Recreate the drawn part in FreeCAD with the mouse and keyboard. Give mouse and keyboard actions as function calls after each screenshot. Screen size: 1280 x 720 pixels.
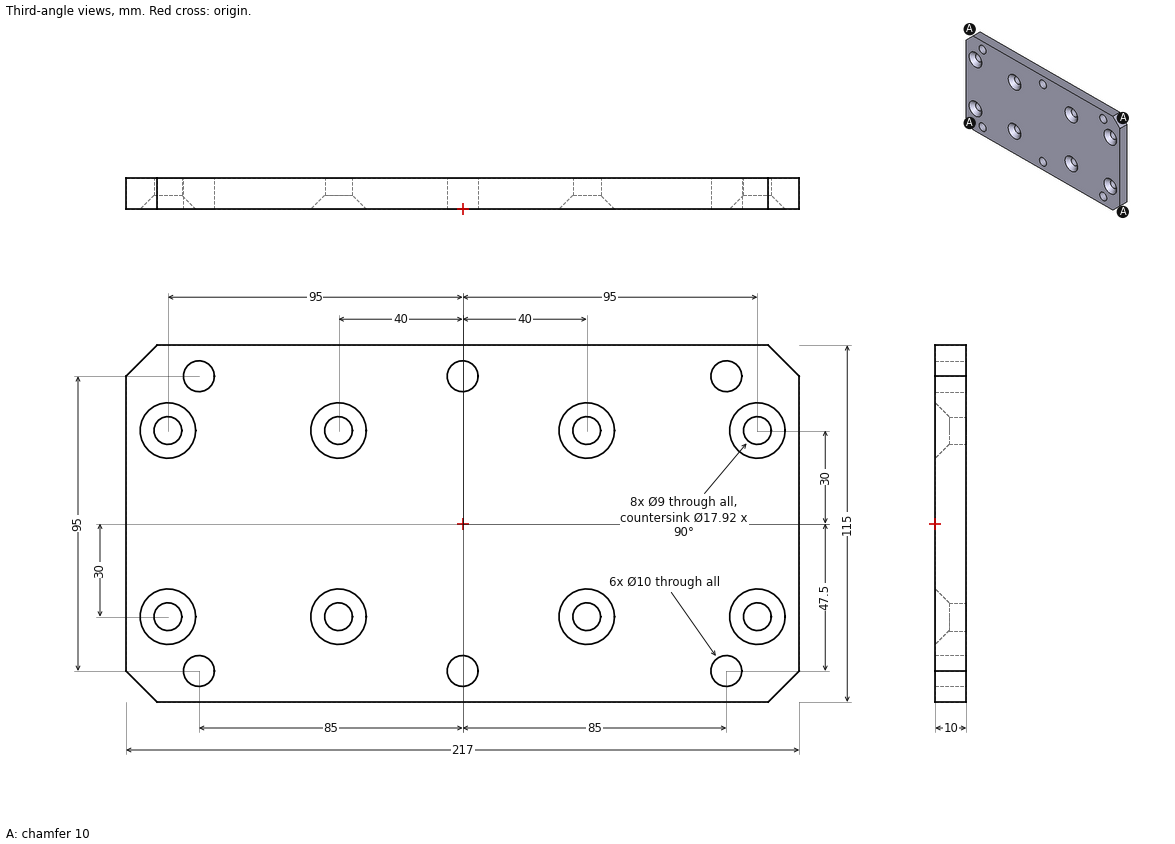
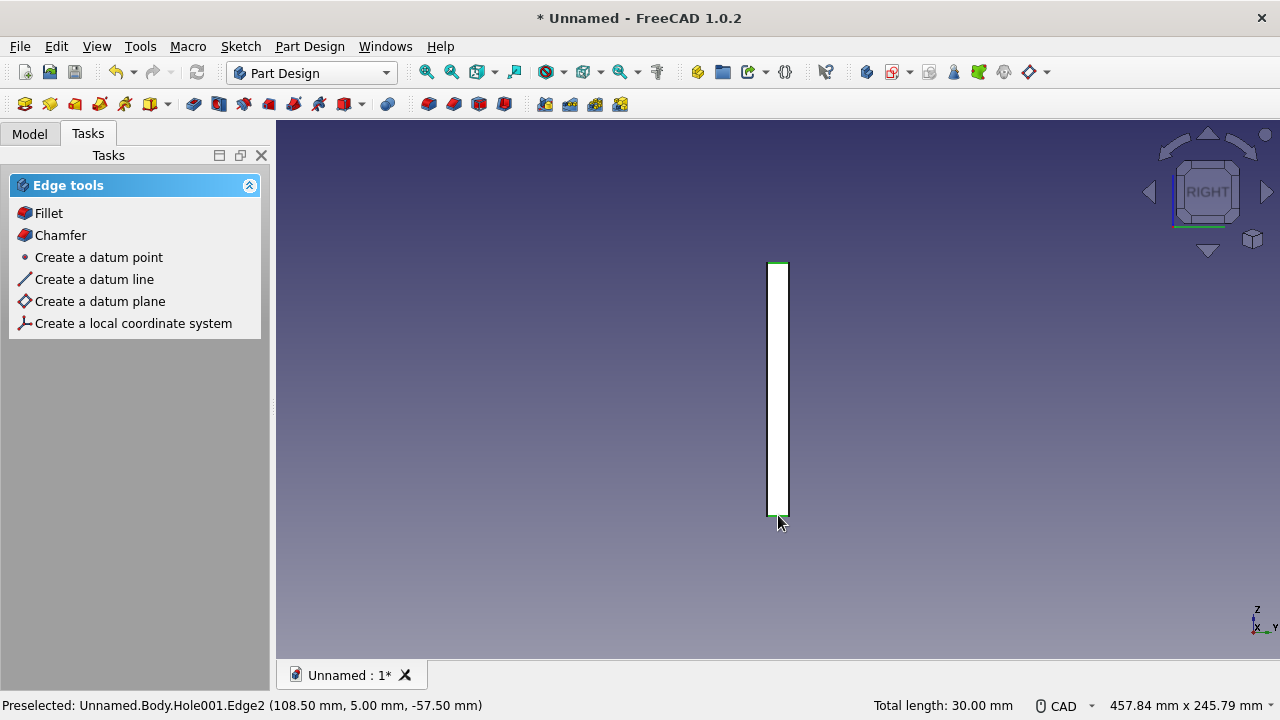
scroll(778, 515, up, 4)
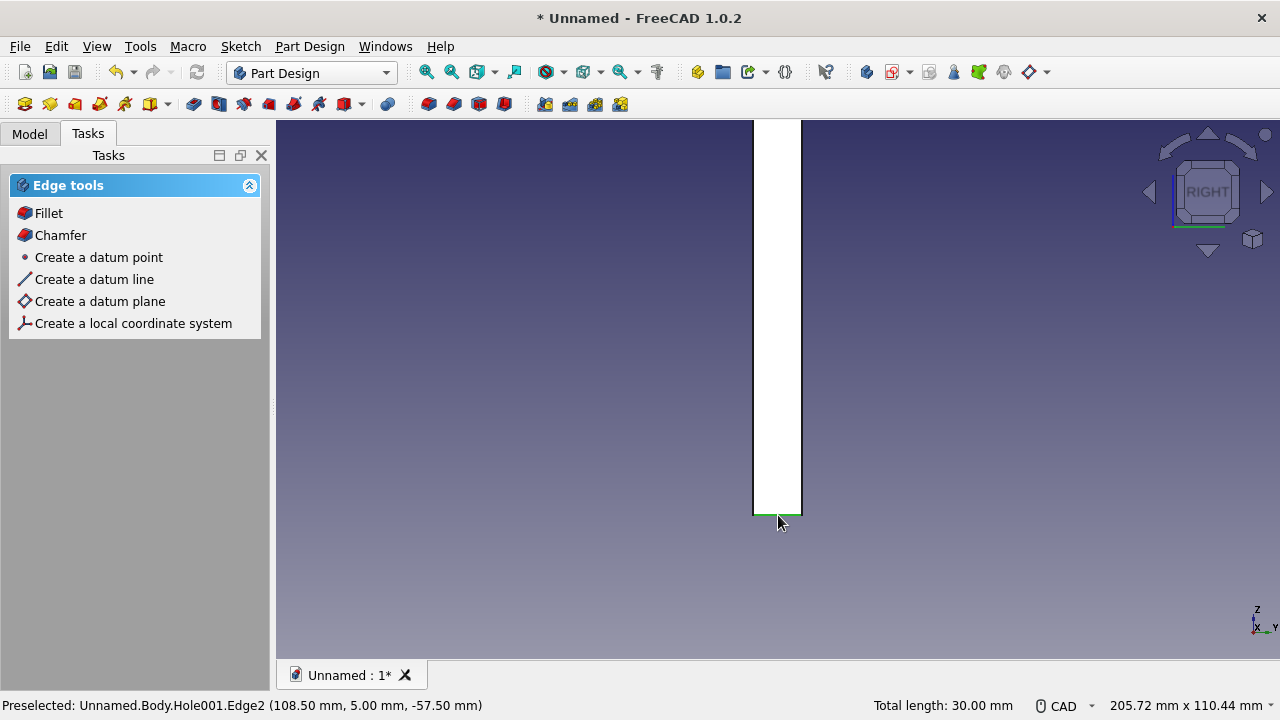
click(427, 72)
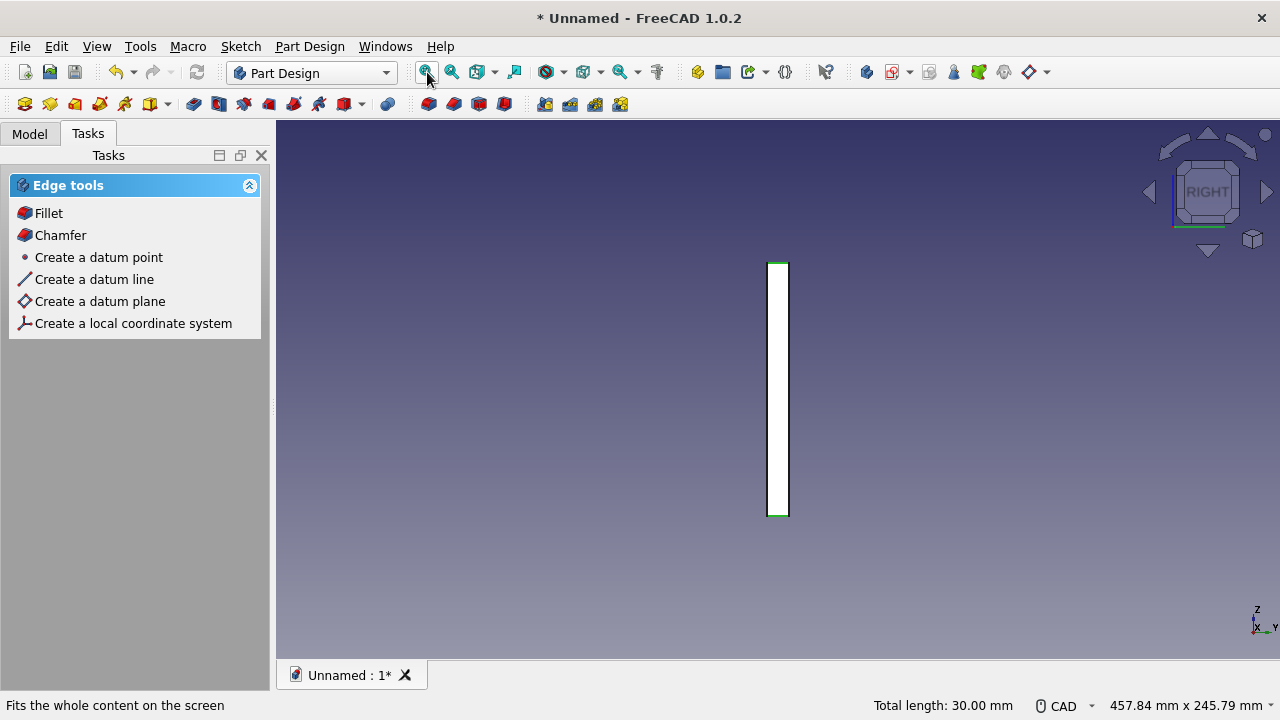
key(5)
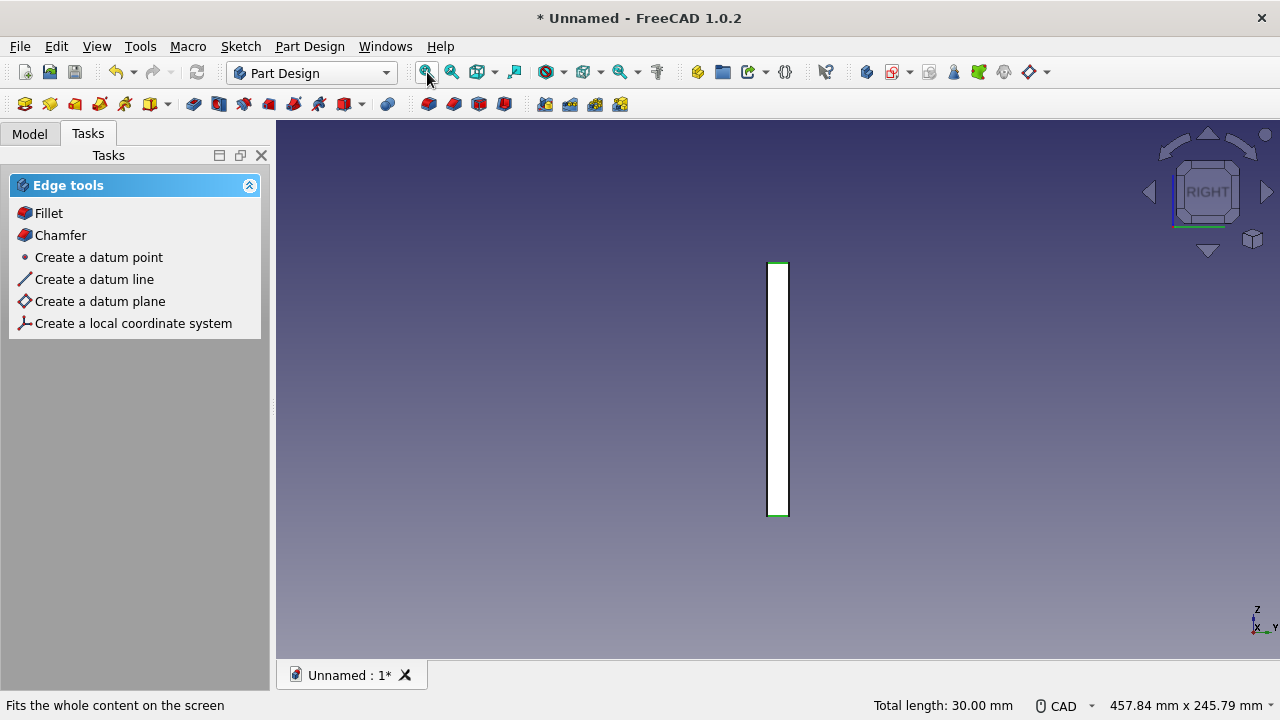
click(540, 388, ctrl)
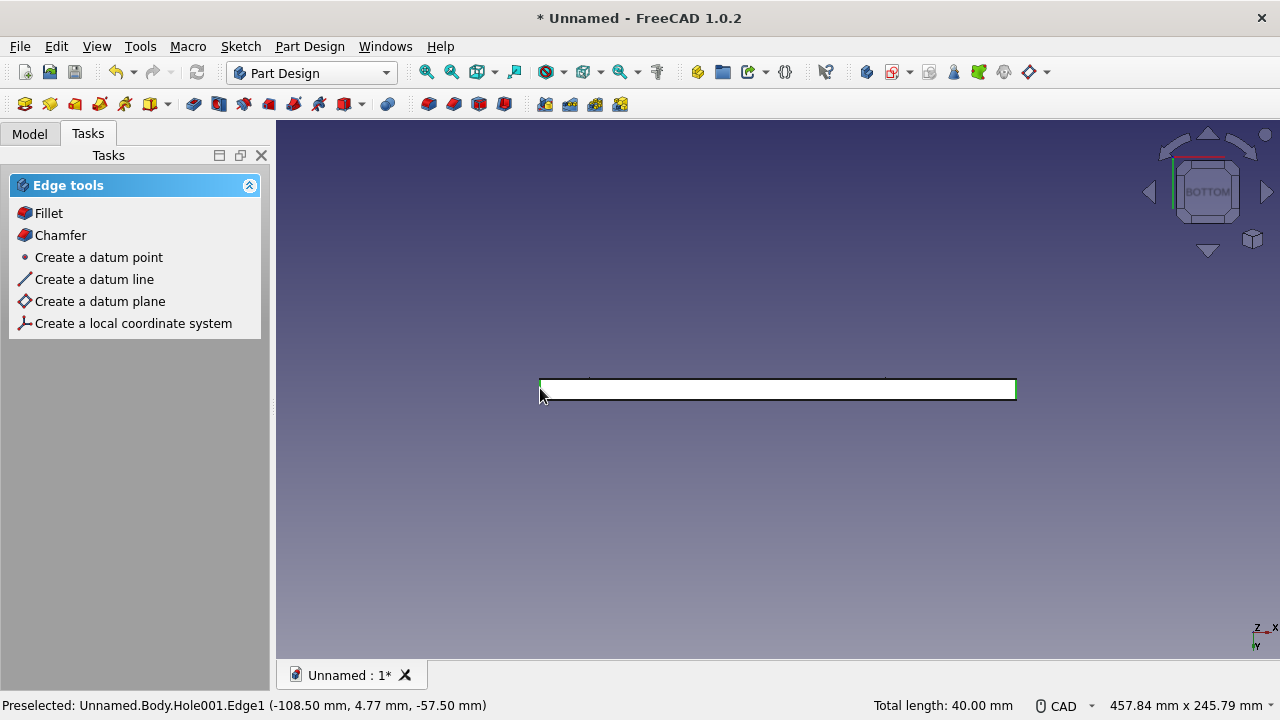
click(454, 104)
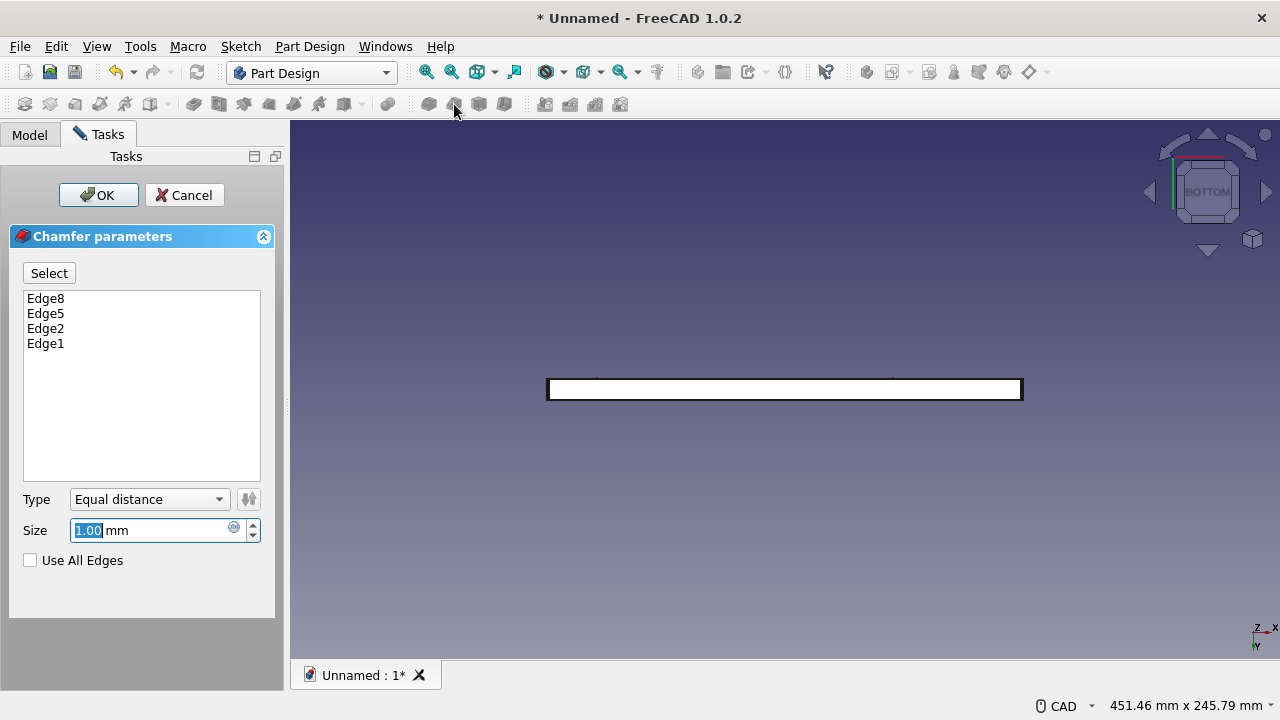
text(10)
key(Tab)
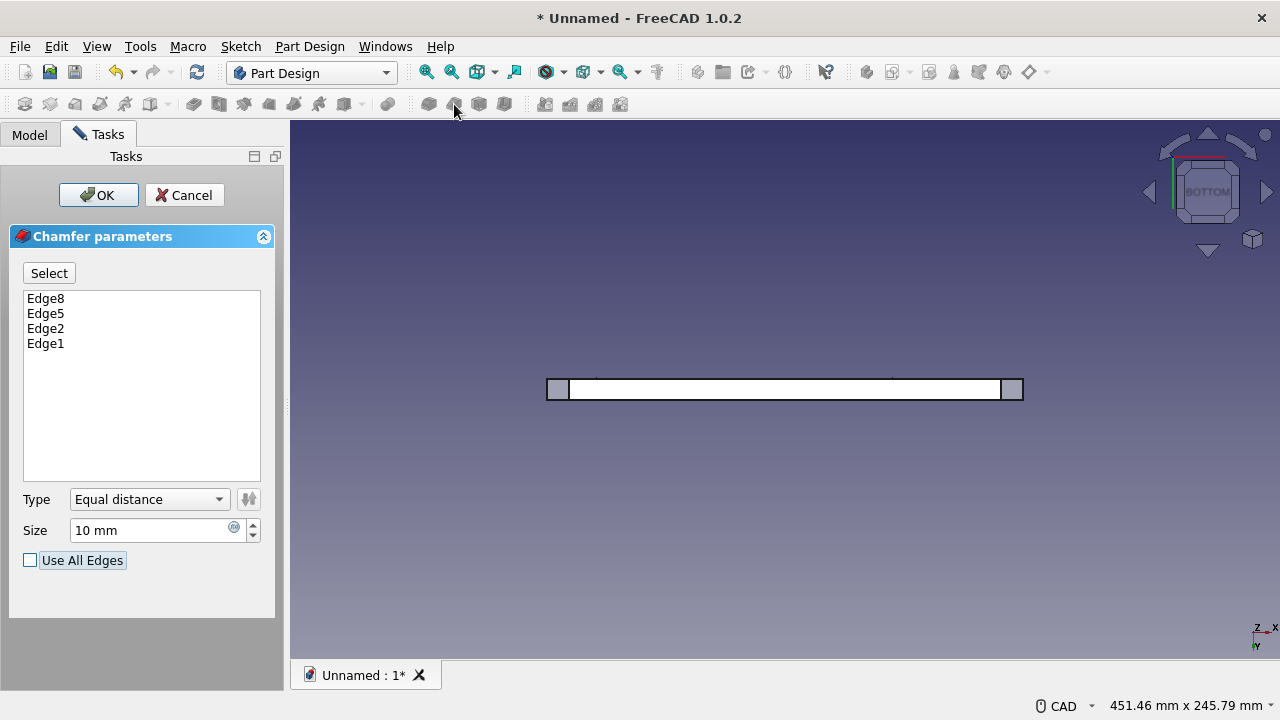
click(99, 195)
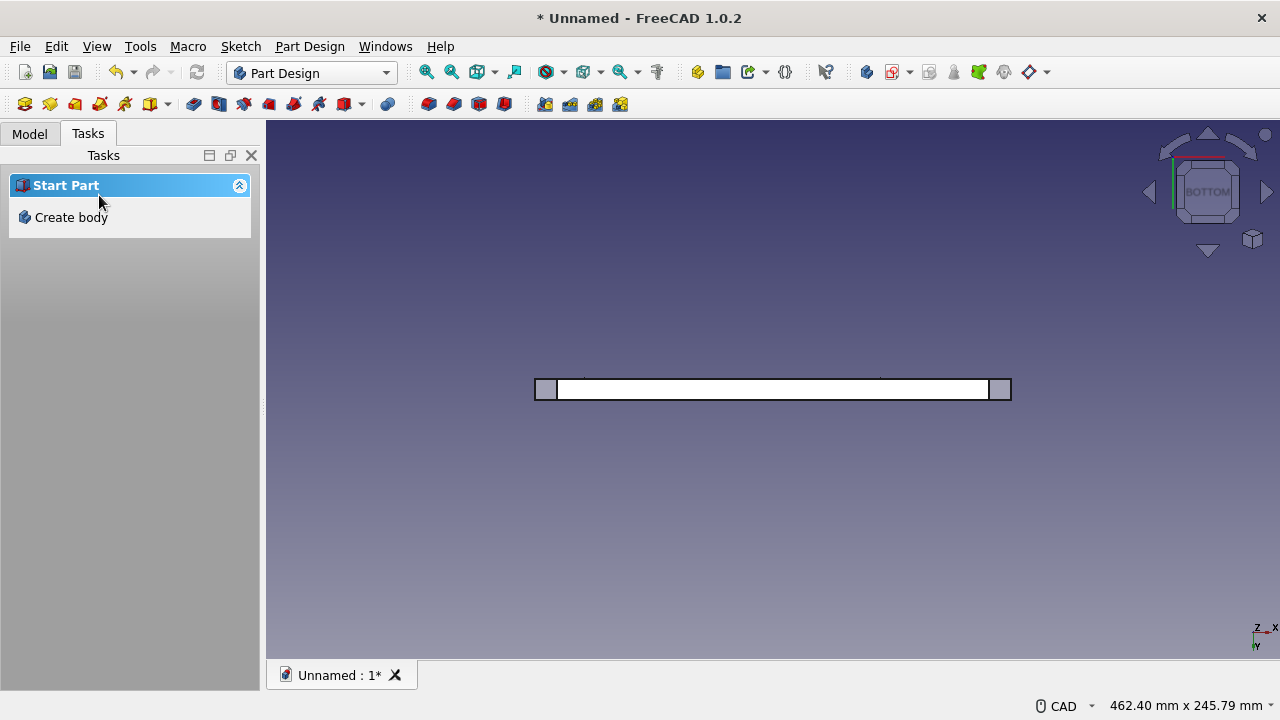
key(0)